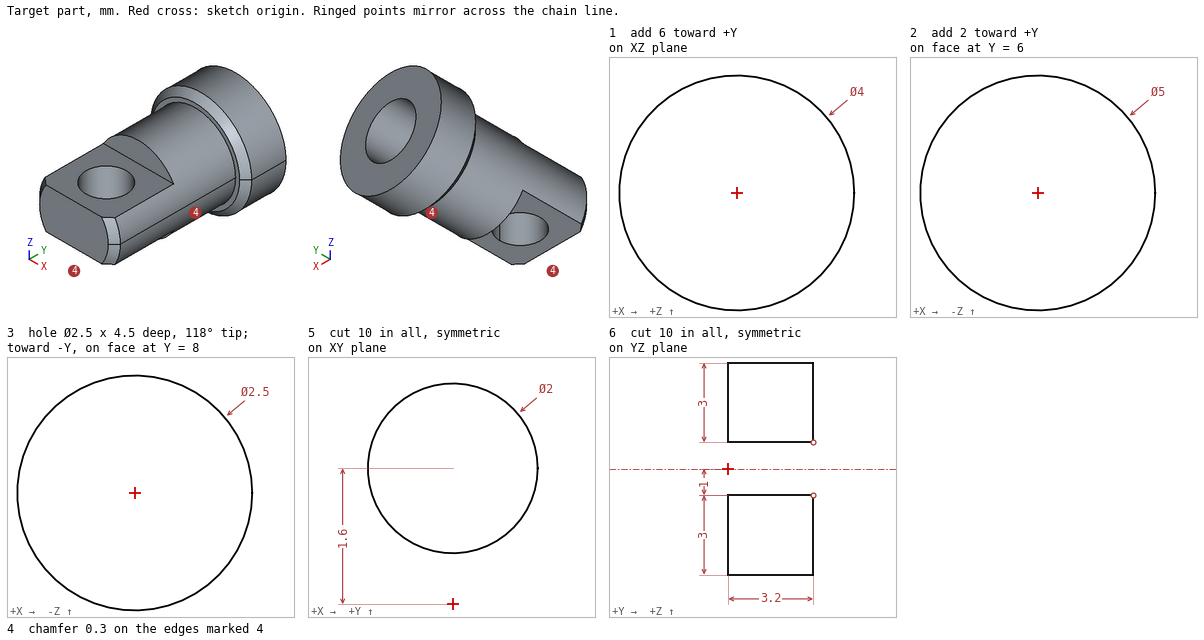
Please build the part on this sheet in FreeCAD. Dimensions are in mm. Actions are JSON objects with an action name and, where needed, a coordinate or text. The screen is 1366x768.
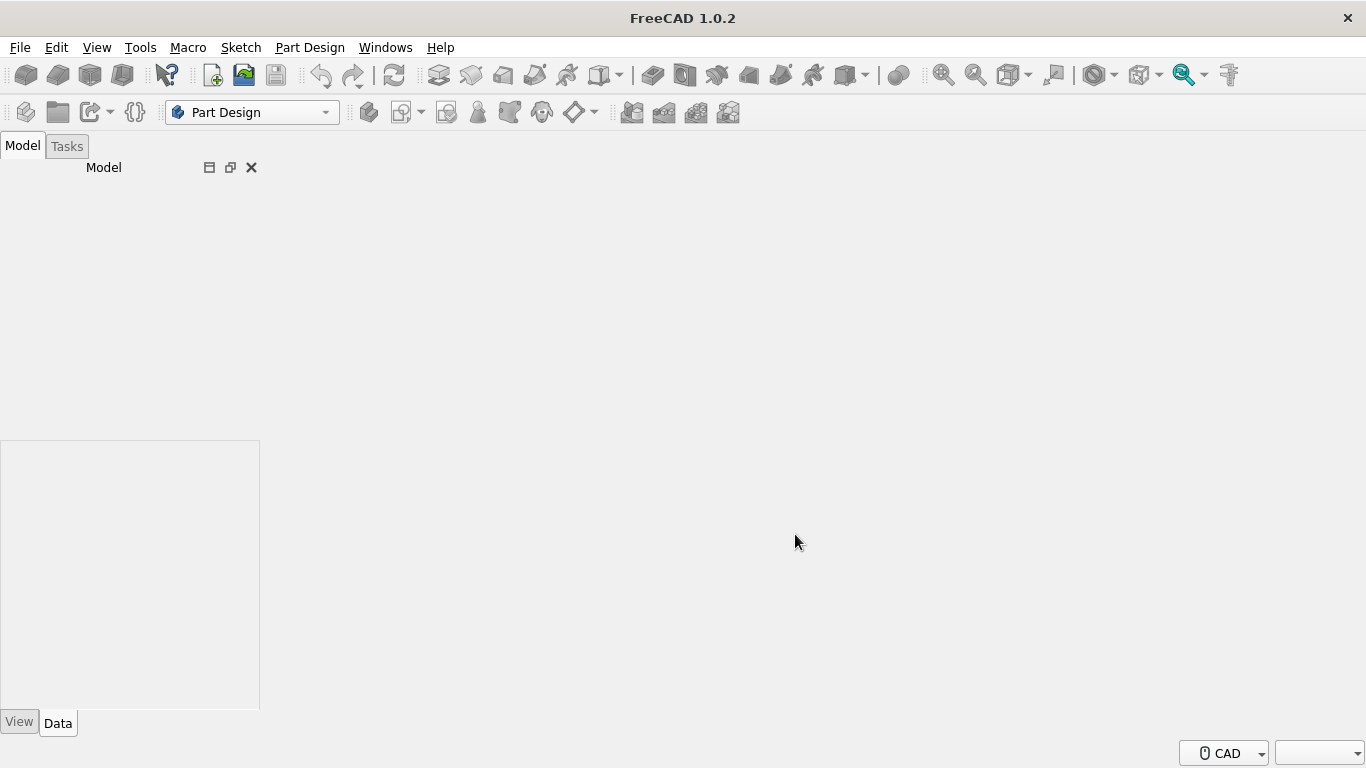
{"action": "left_click", "coordinate": [212, 76]}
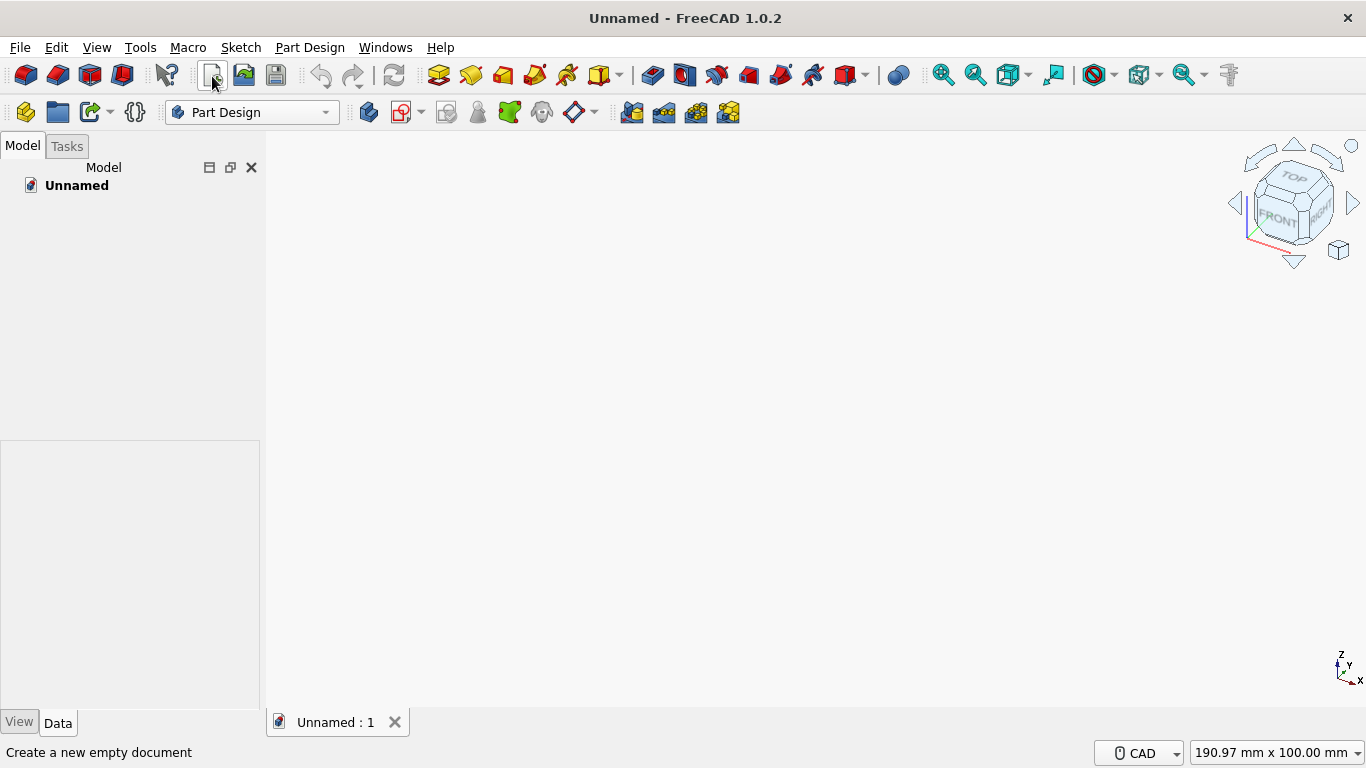
{"action": "left_click", "coordinate": [402, 112]}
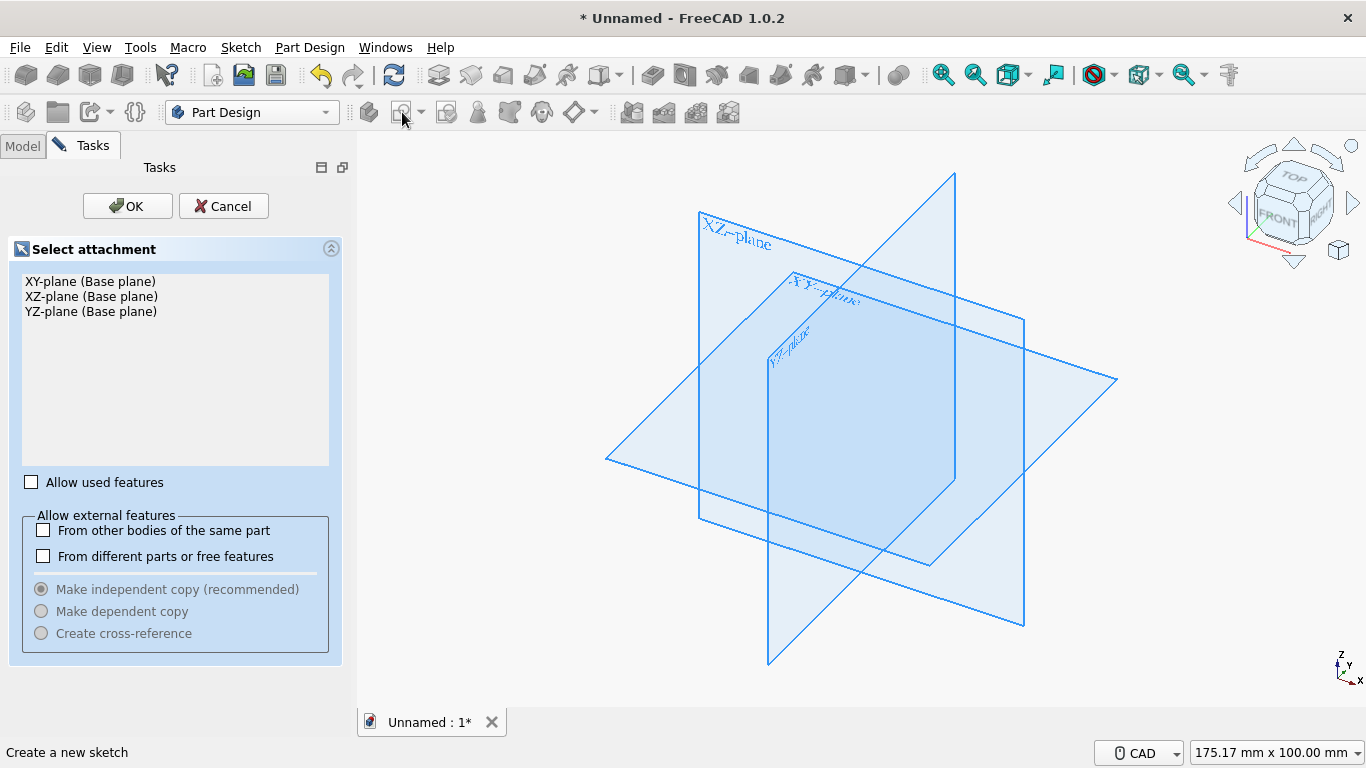
{"action": "left_click", "coordinate": [82, 296]}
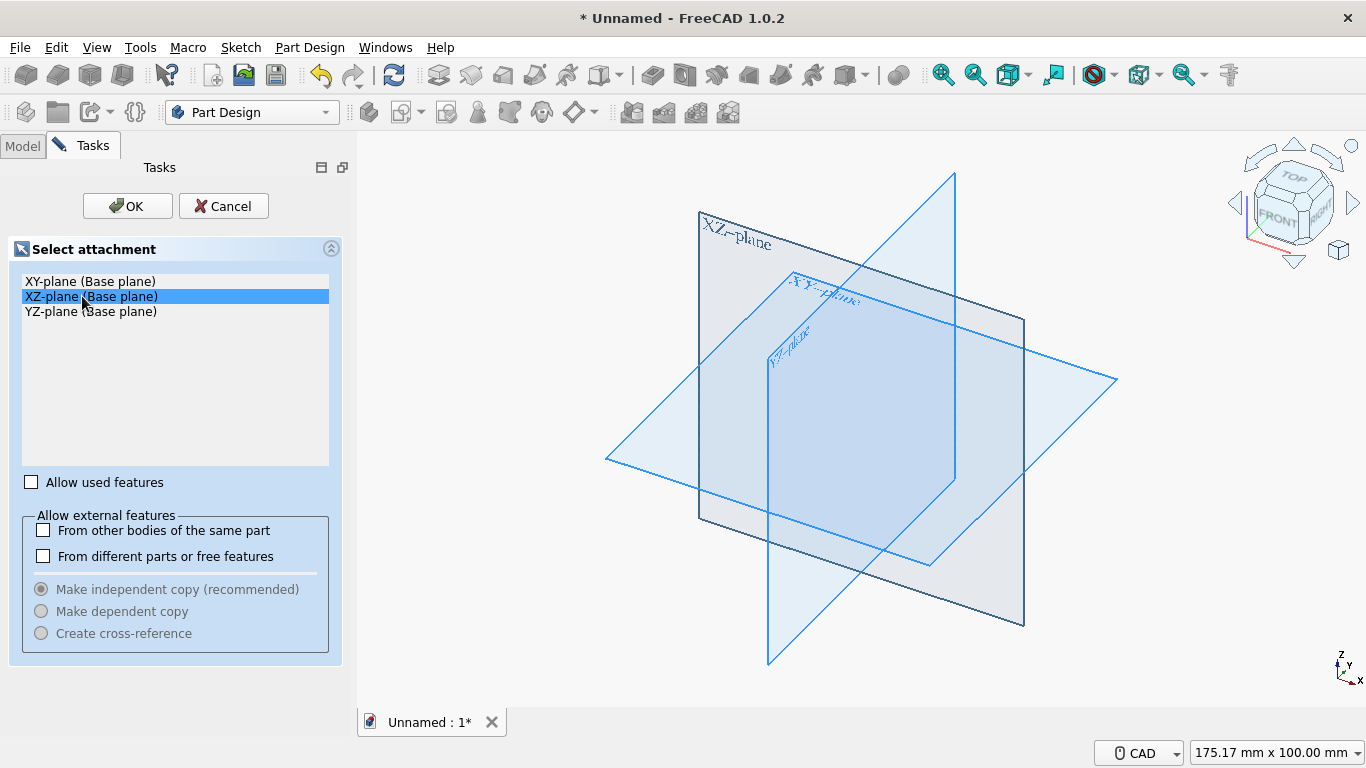
{"action": "left_click", "coordinate": [128, 206]}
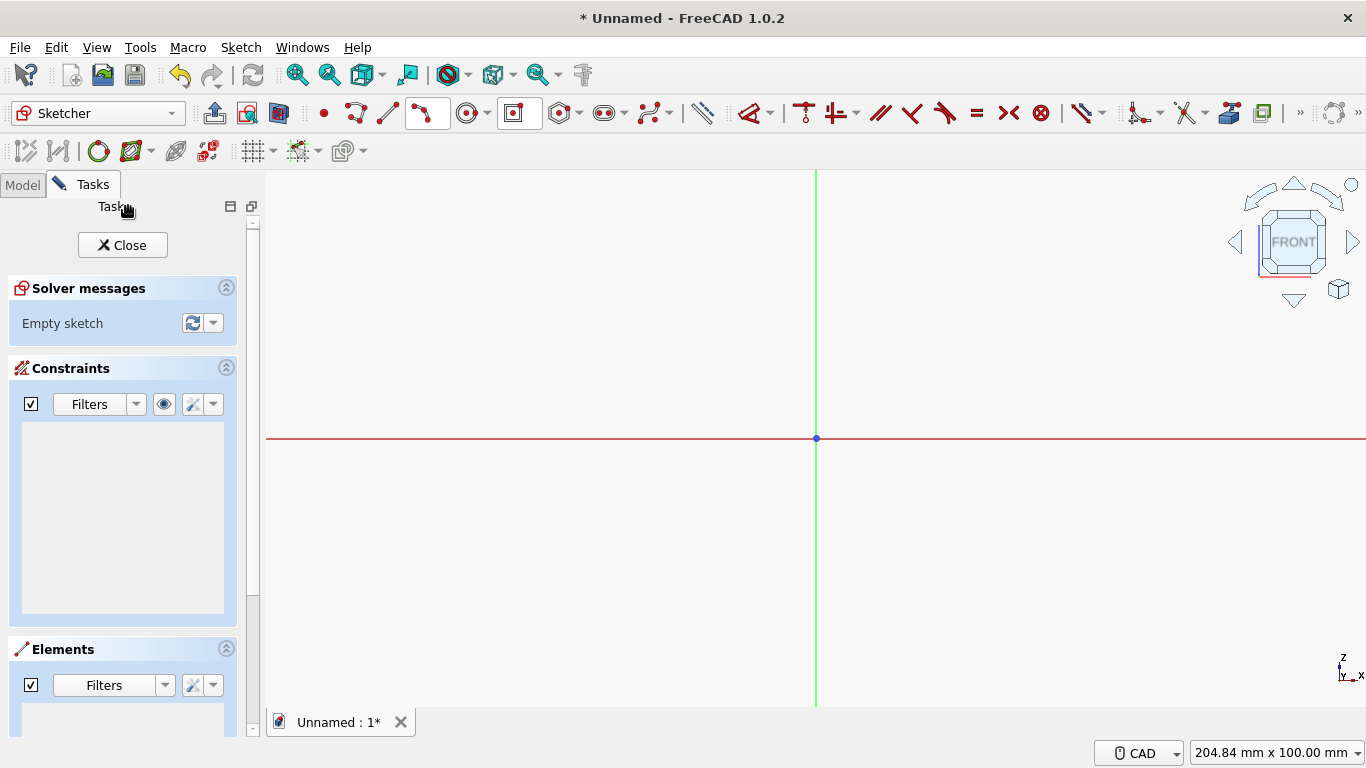
{"action": "scroll", "coordinate": [820, 438], "scroll_direction": "up", "scroll_amount": 14}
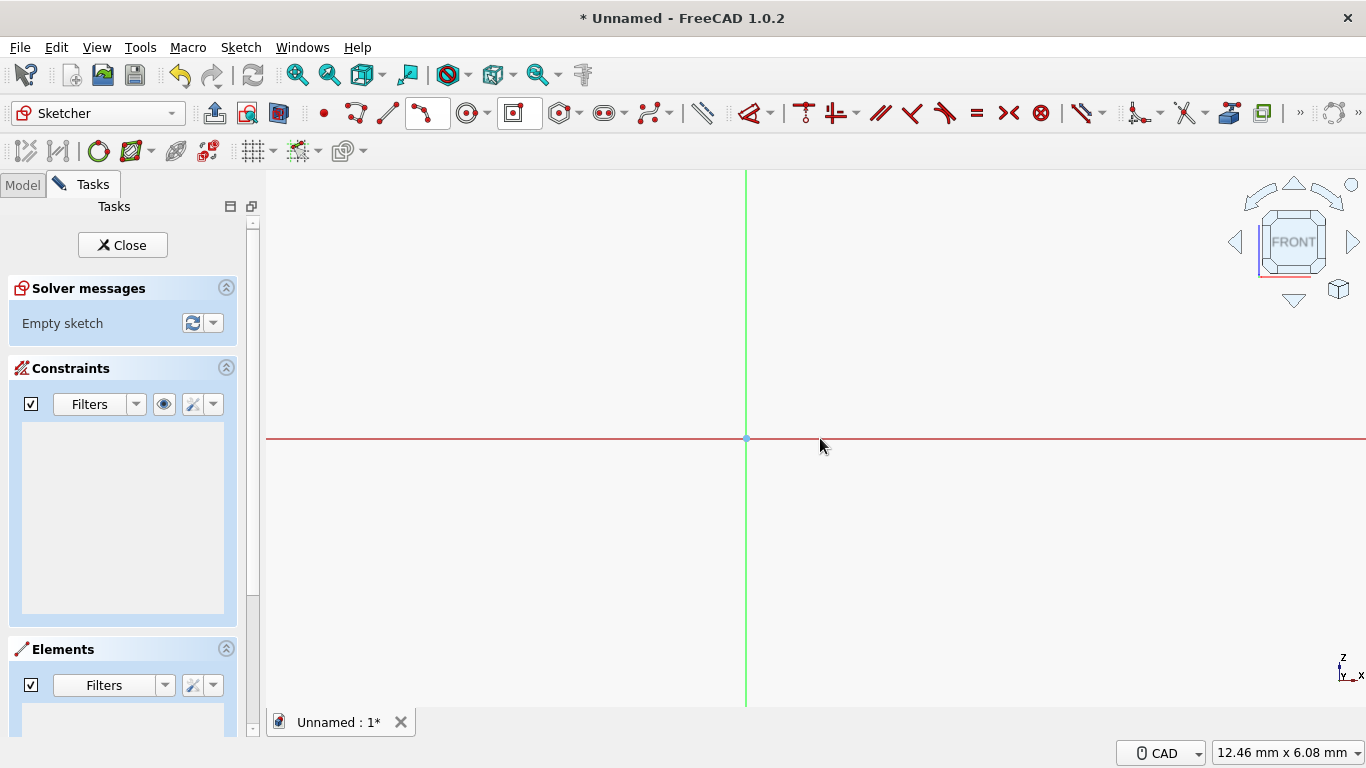
{"action": "key", "text": "g c"}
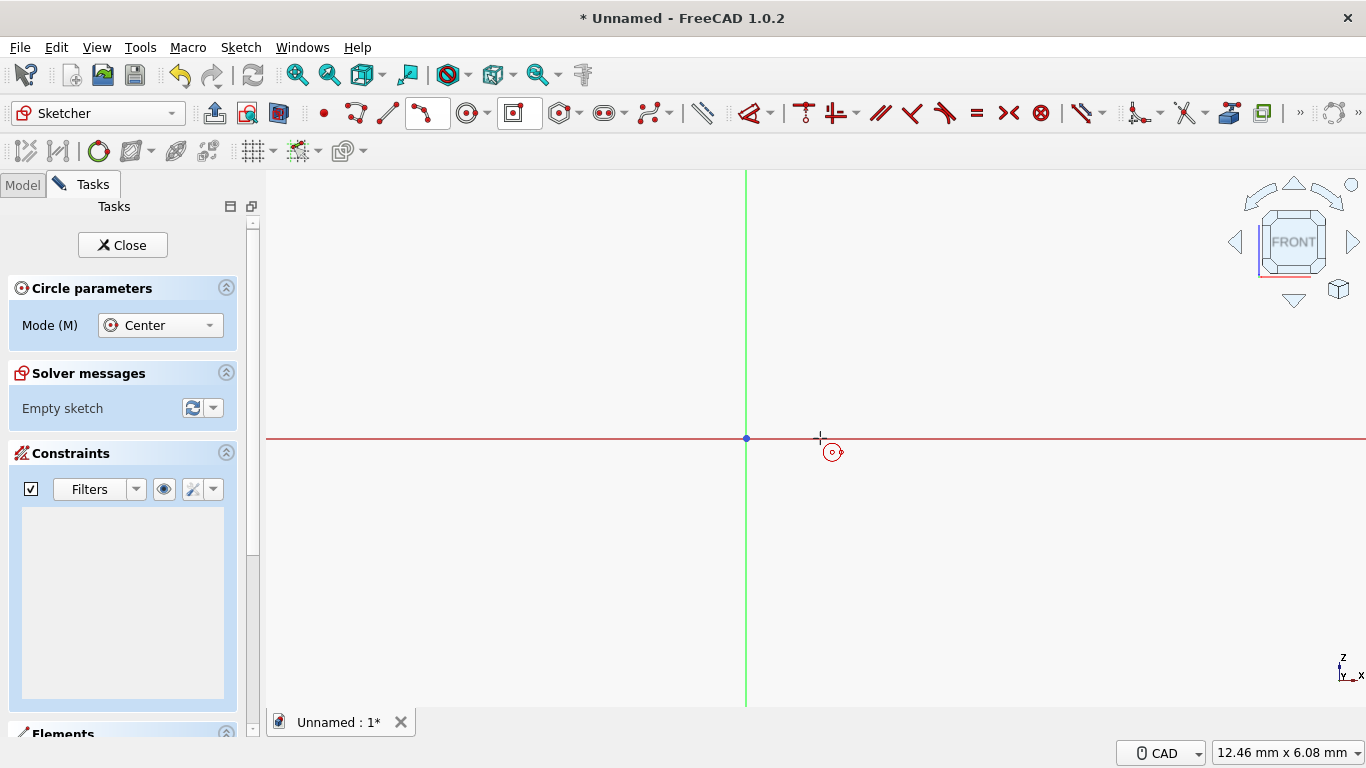
{"action": "left_click", "coordinate": [746, 438]}
{"action": "left_click", "coordinate": [871, 314]}
{"action": "key", "text": "Escape"}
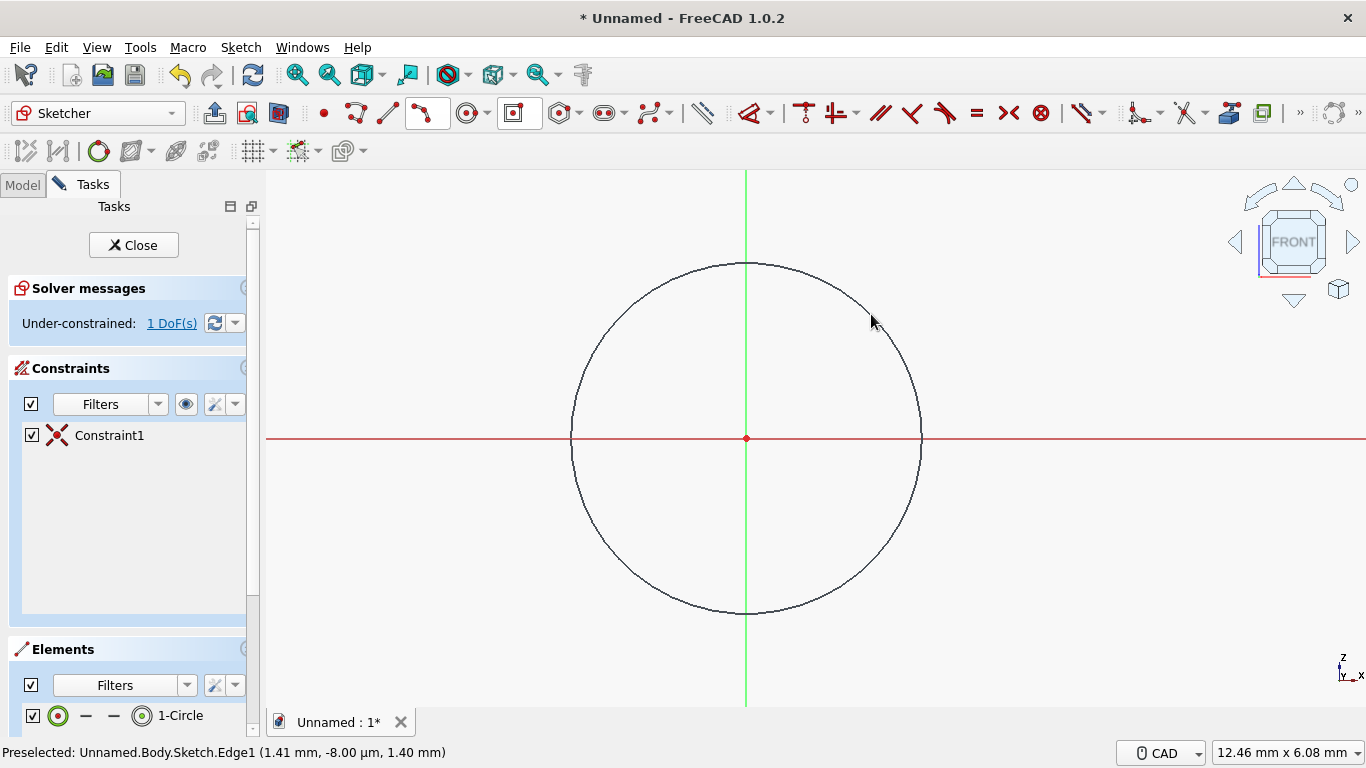
{"action": "left_click", "coordinate": [870, 314]}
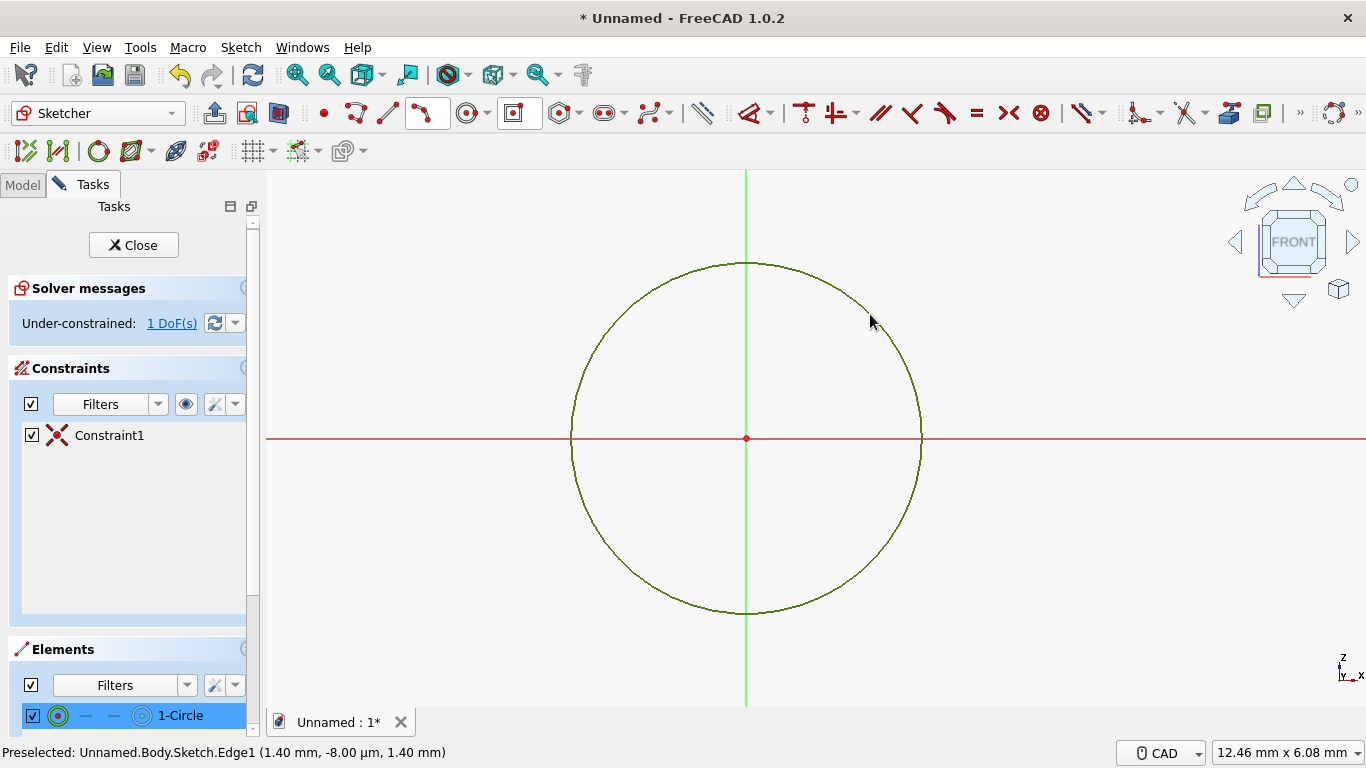
{"action": "key", "text": "k o"}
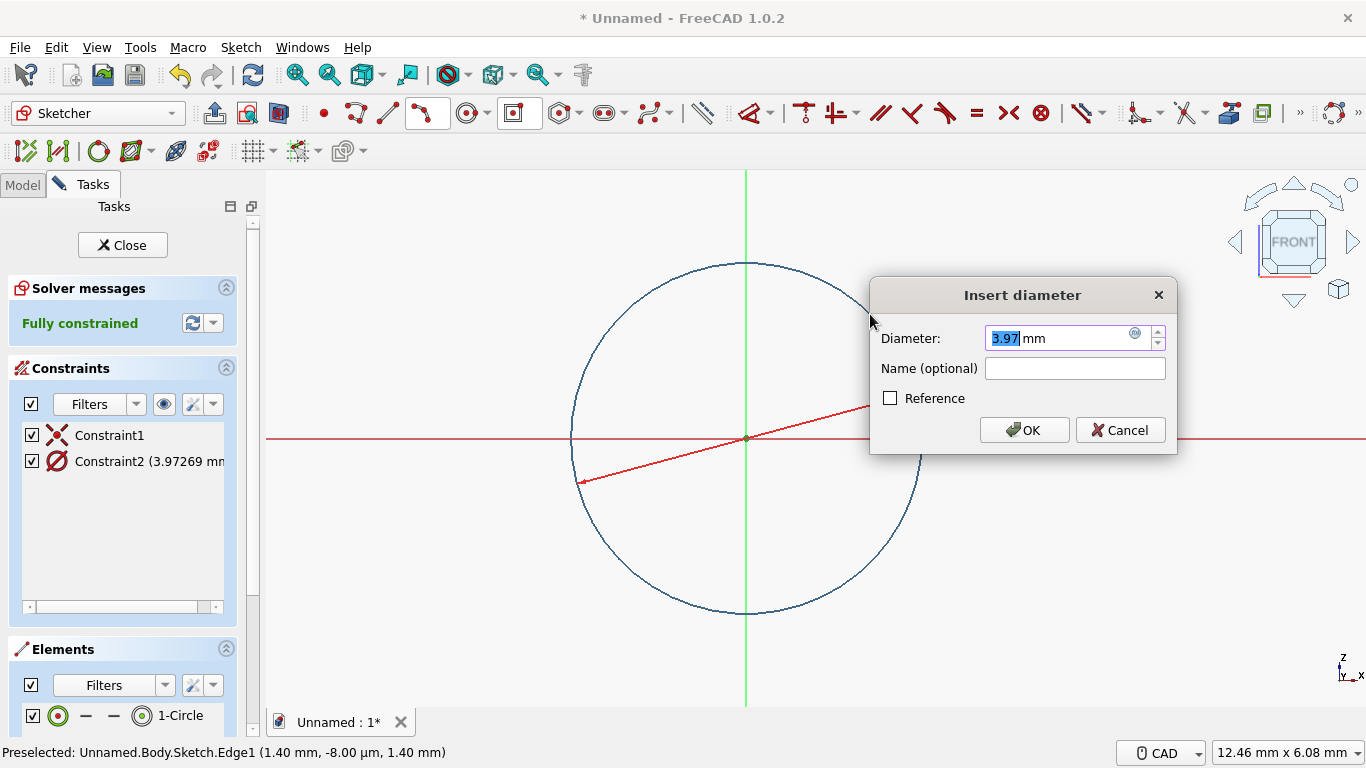
{"action": "type", "text": "4"}
{"action": "key", "text": "Return"}